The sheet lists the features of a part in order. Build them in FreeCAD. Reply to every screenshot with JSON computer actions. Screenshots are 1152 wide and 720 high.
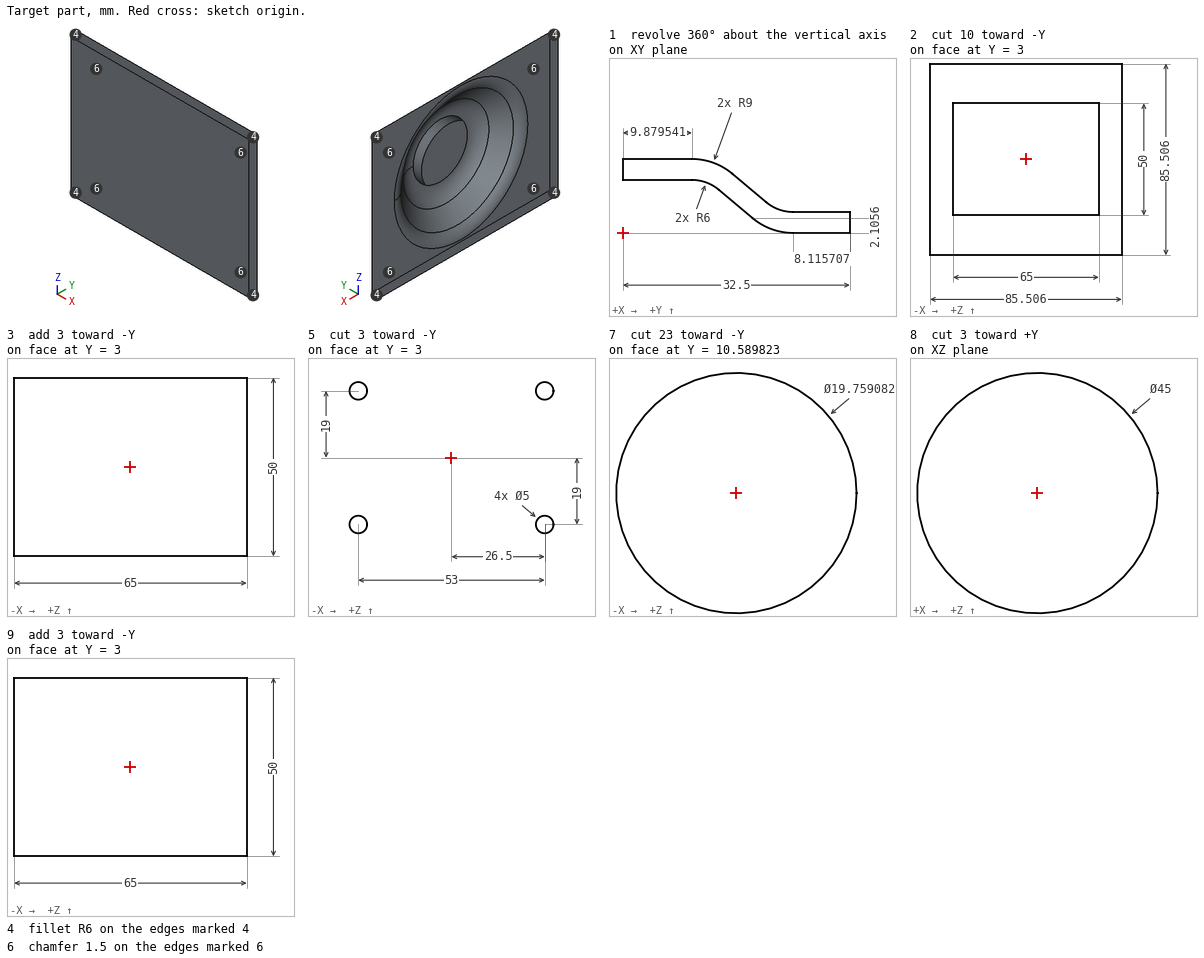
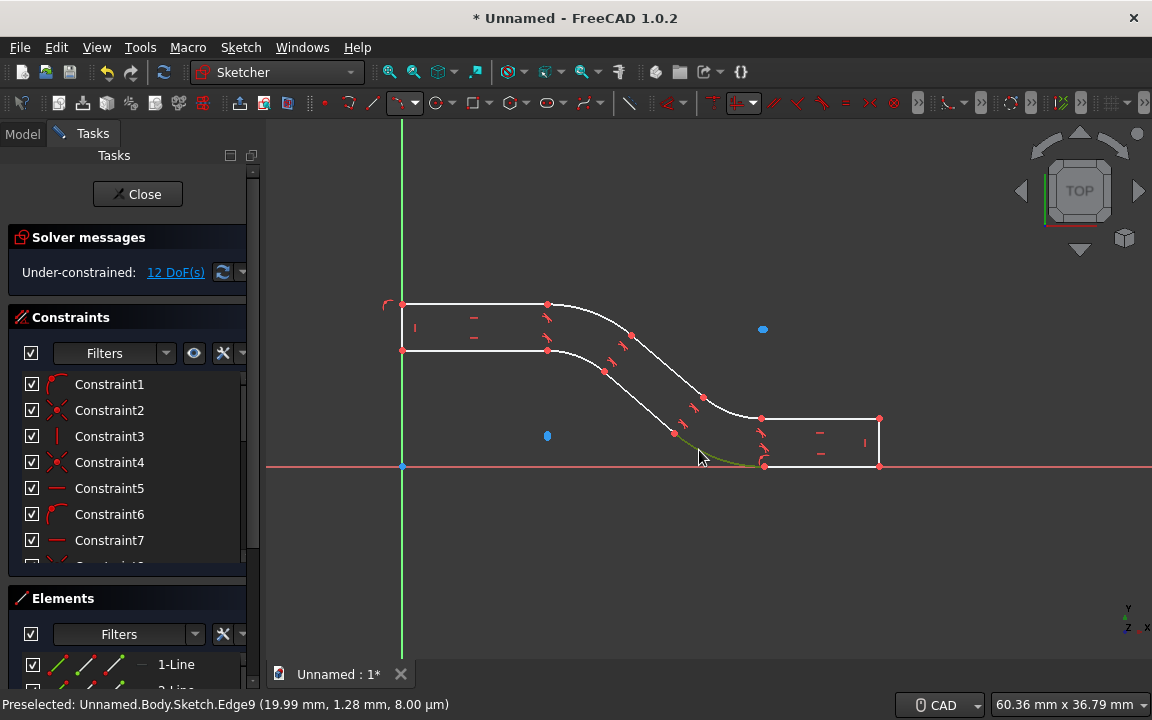
{"action": "left_click", "coordinate": [719, 408]}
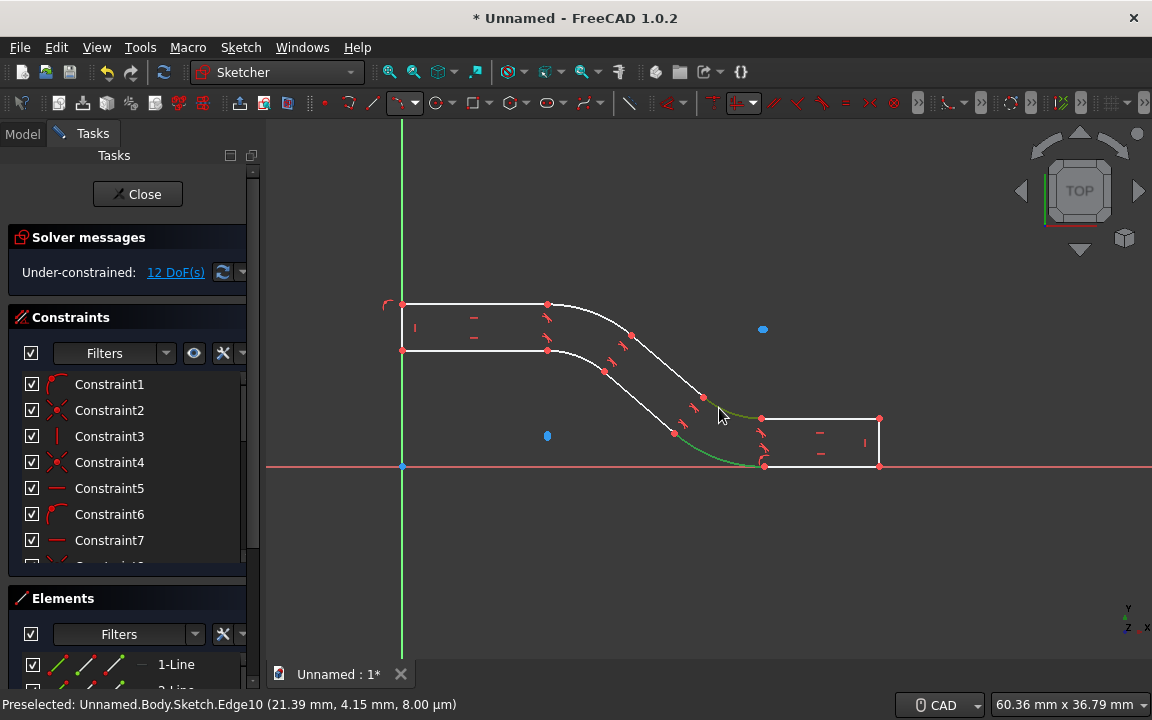
{"action": "left_click", "coordinate": [714, 104]}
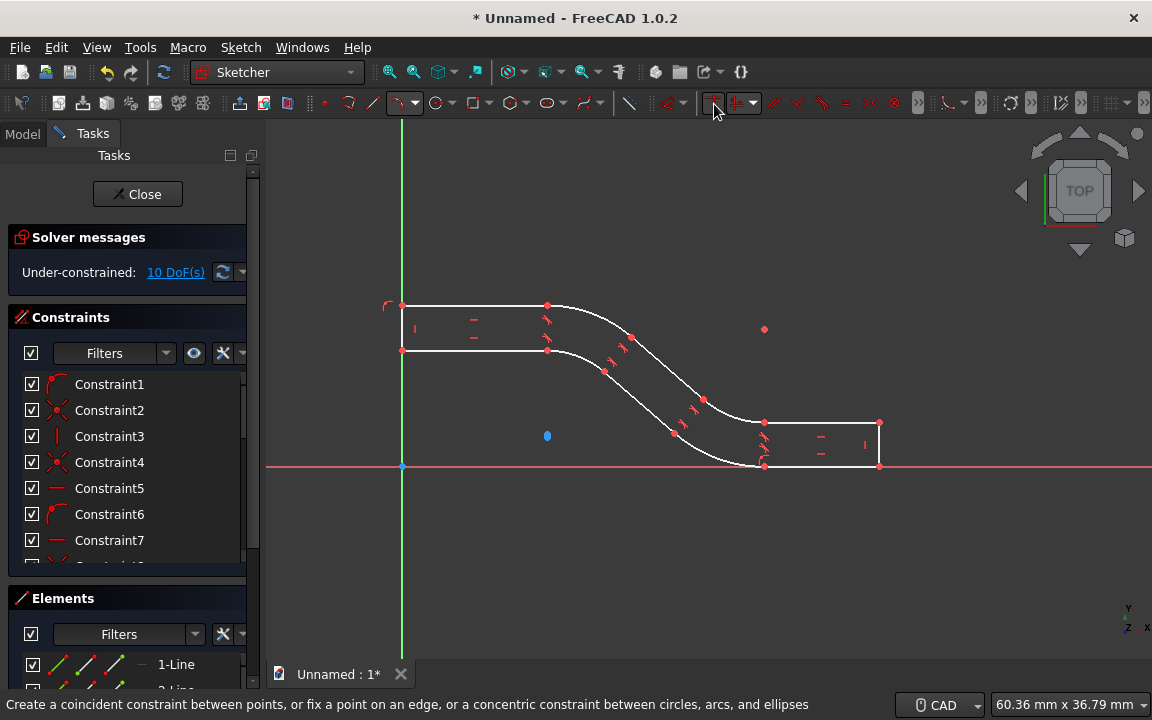
{"action": "left_click", "coordinate": [609, 321]}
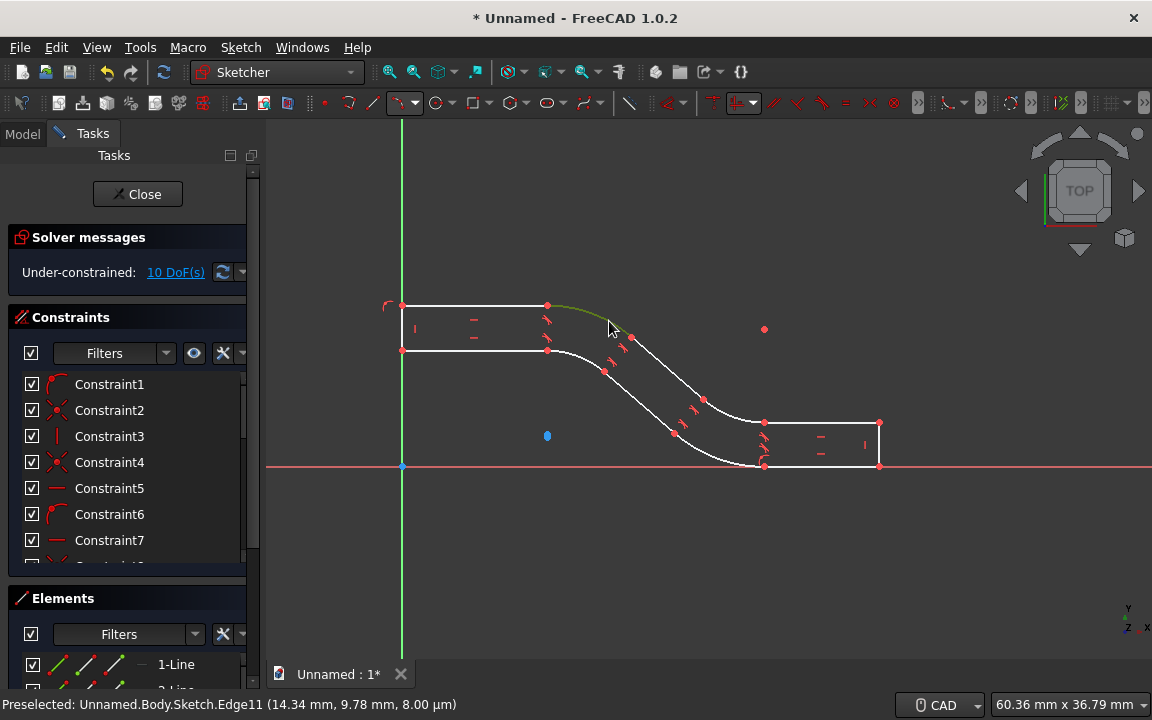
{"action": "left_click", "coordinate": [589, 361]}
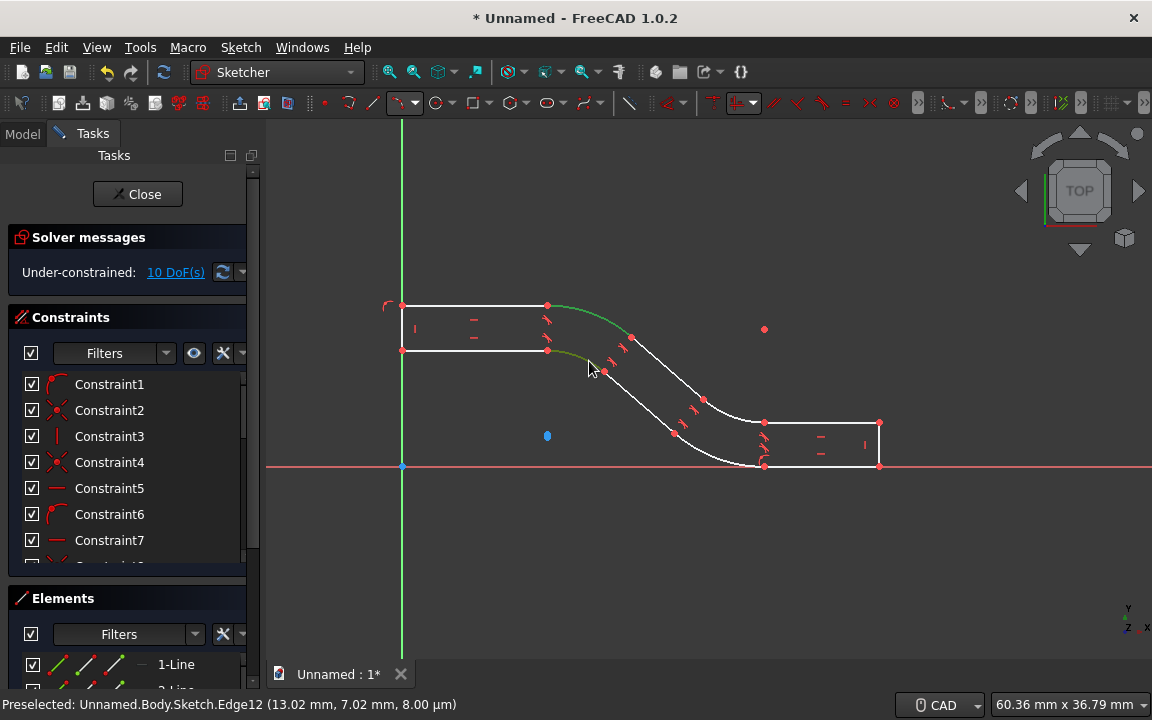
{"action": "left_click", "coordinate": [714, 104]}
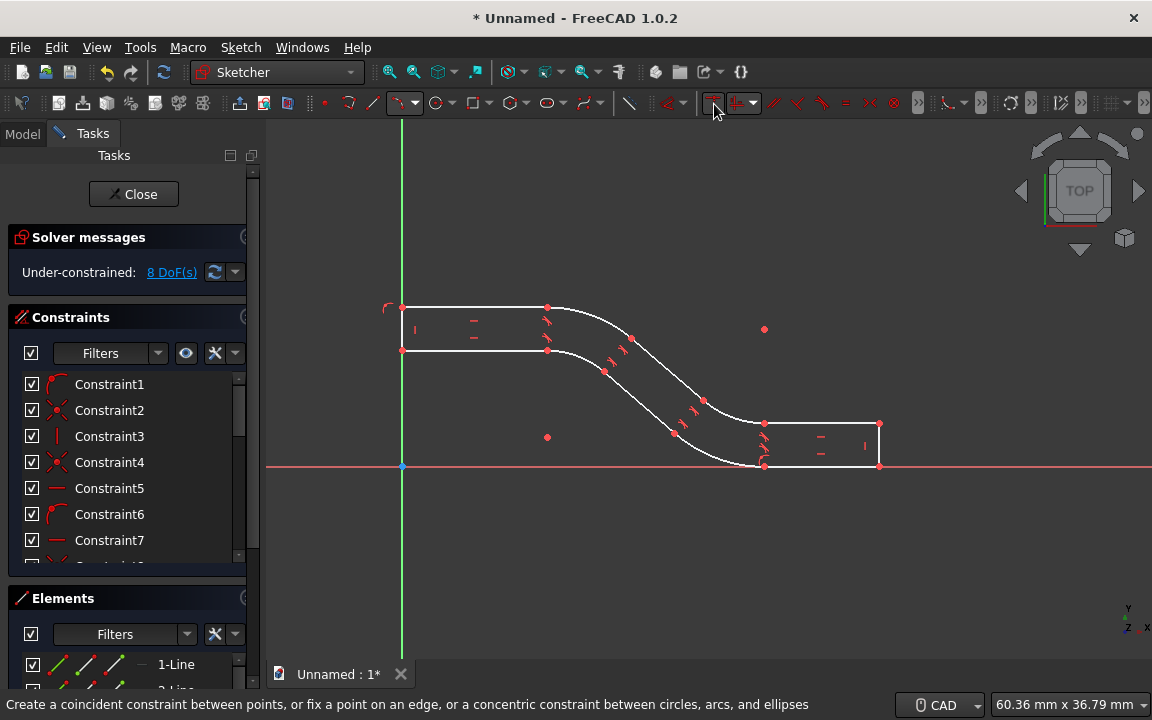
{"action": "left_click", "coordinate": [699, 450]}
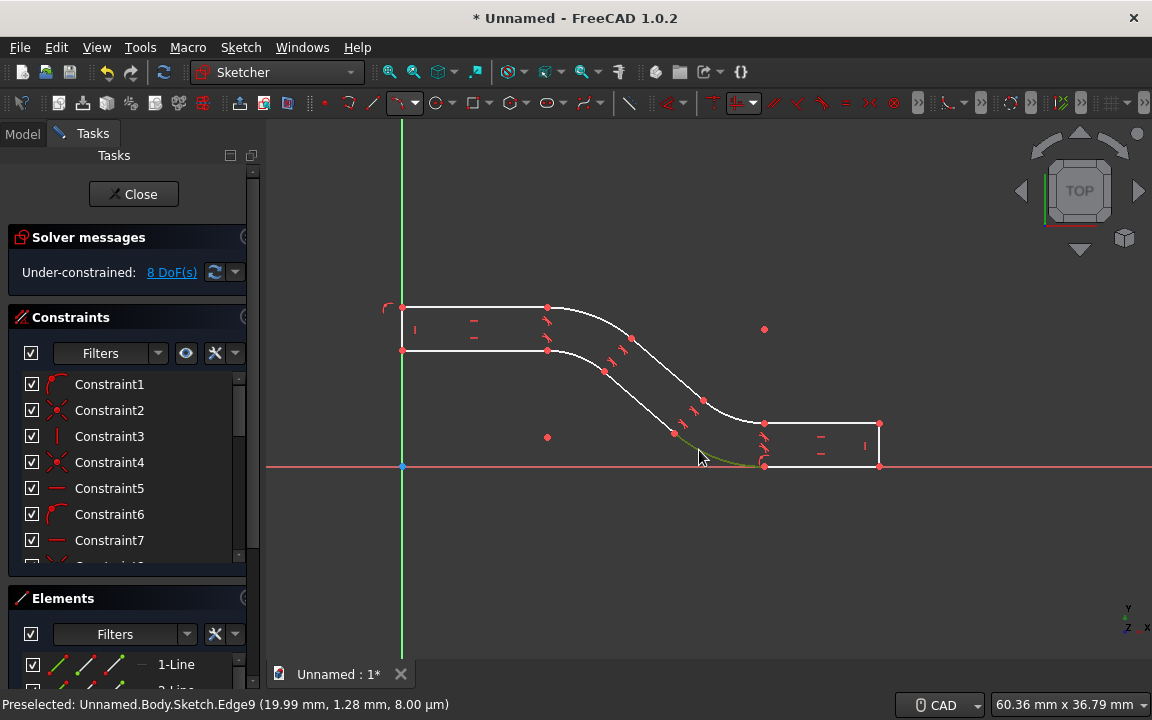
{"action": "left_click", "coordinate": [609, 323]}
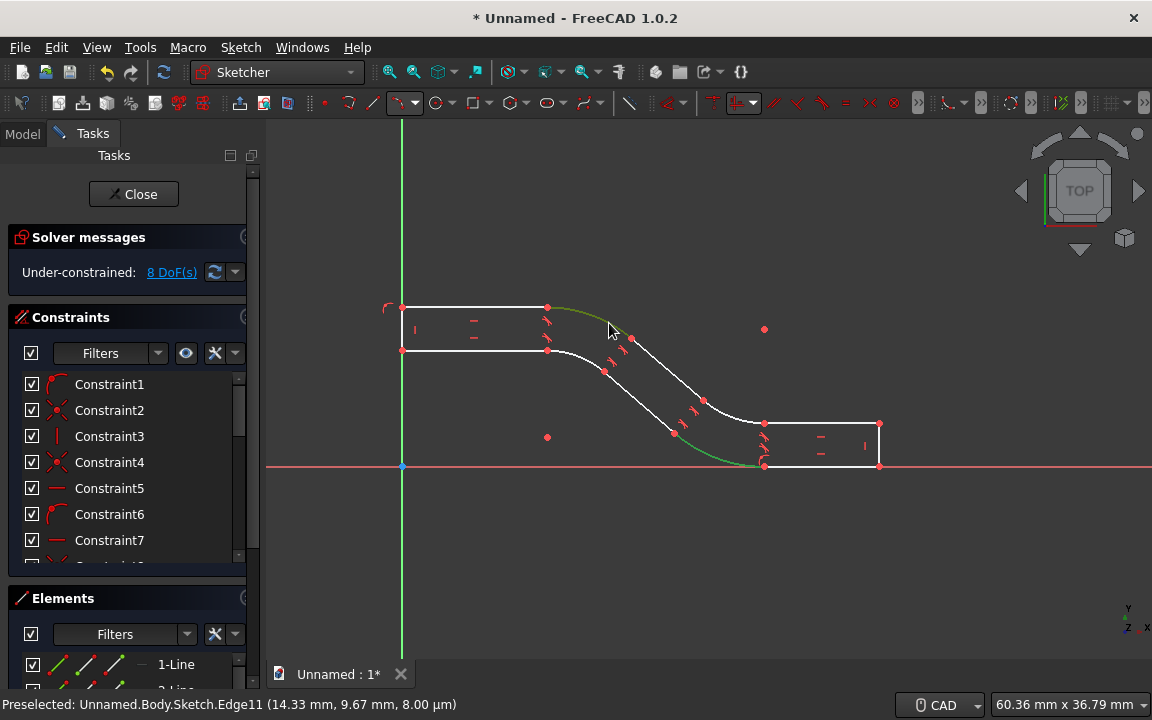
{"action": "left_click", "coordinate": [846, 104]}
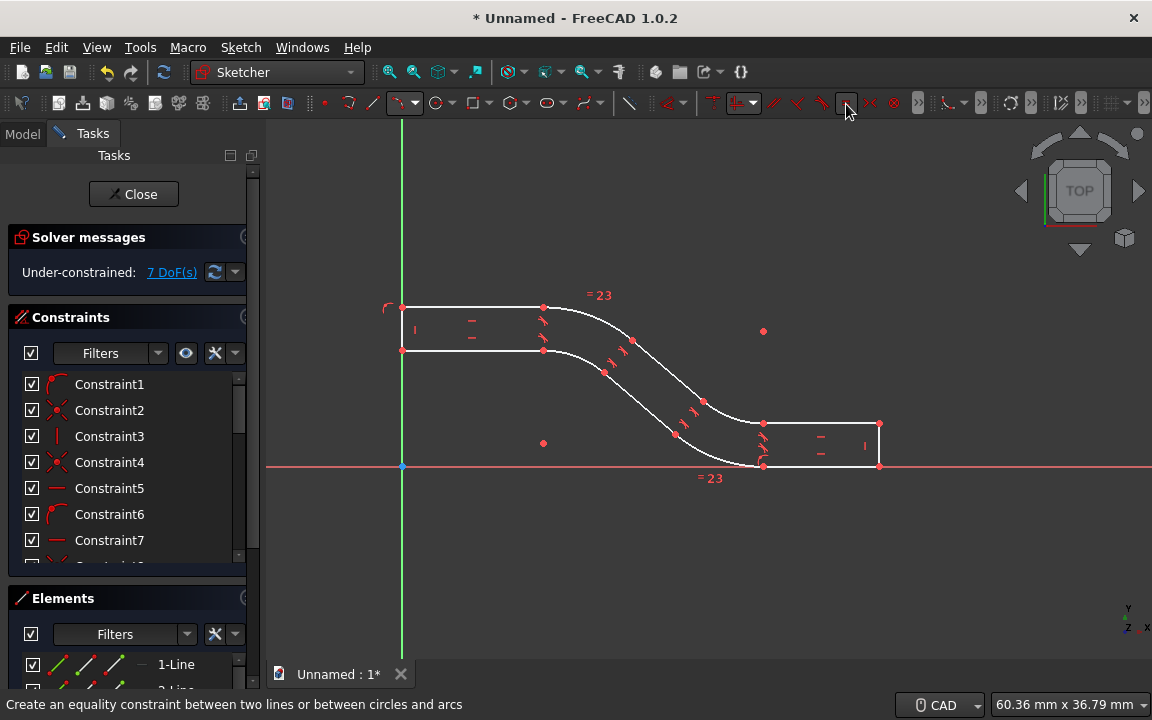
{"action": "left_click", "coordinate": [720, 412]}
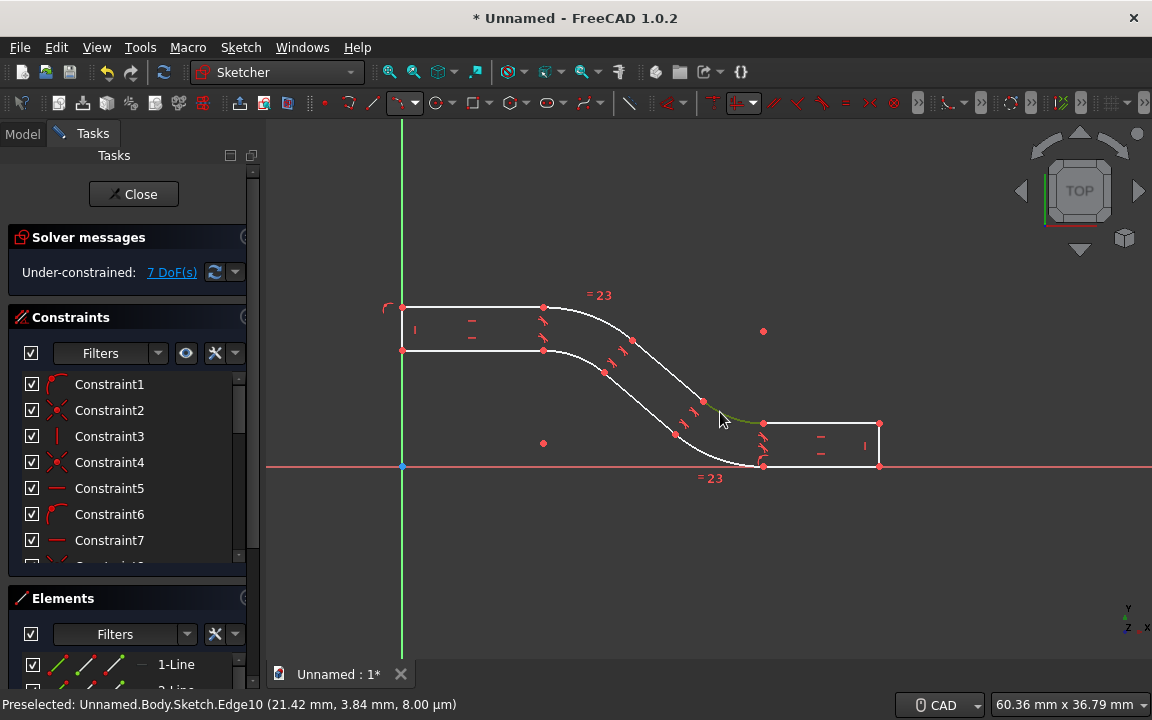
{"action": "left_click", "coordinate": [588, 362]}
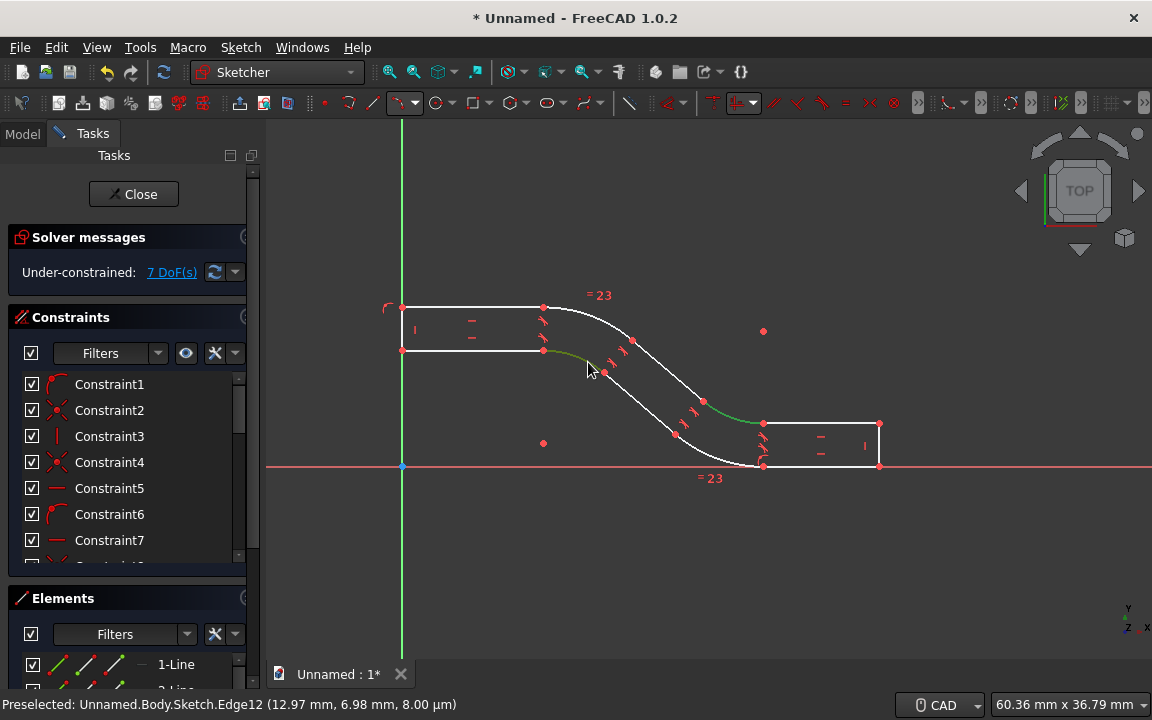
{"action": "left_click", "coordinate": [846, 104]}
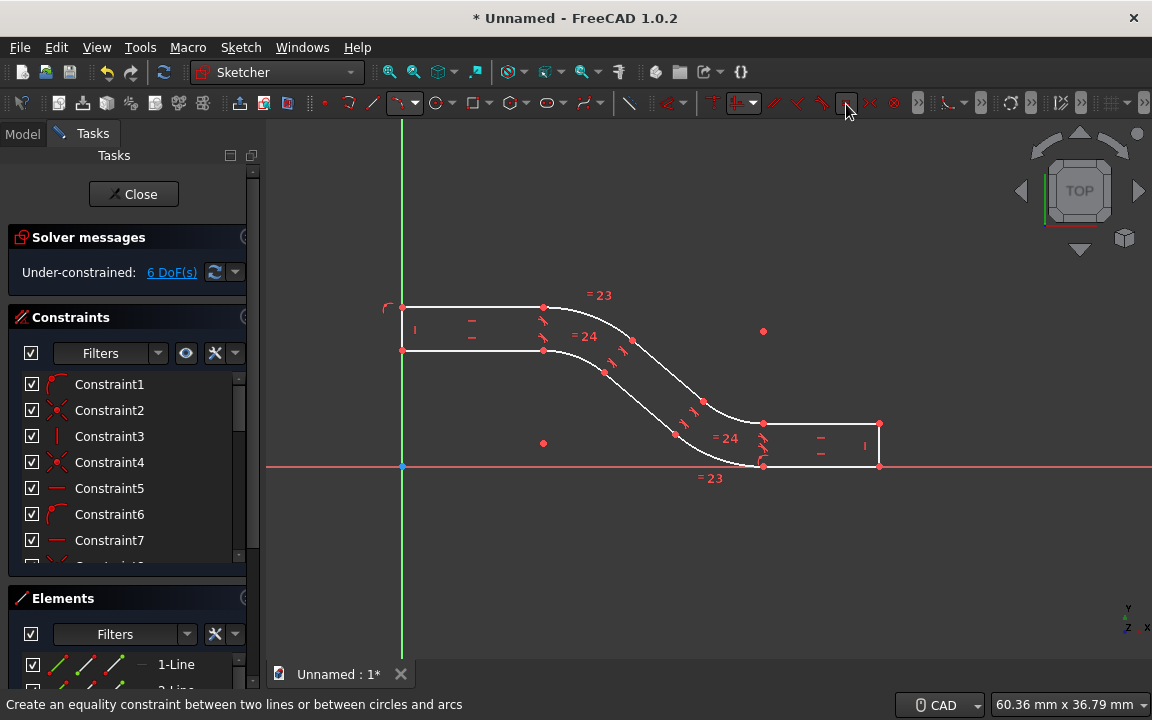
{"action": "left_click", "coordinate": [668, 104]}